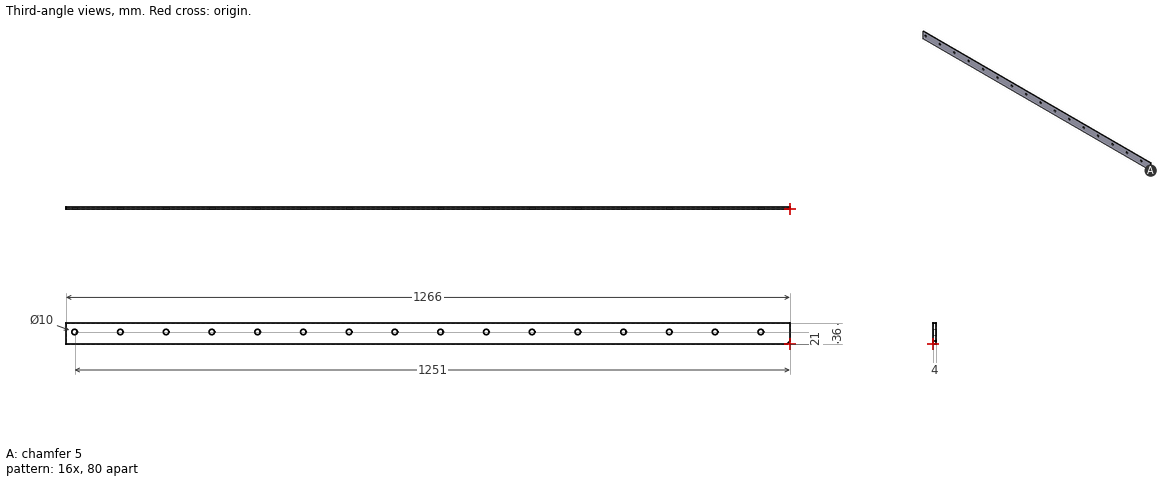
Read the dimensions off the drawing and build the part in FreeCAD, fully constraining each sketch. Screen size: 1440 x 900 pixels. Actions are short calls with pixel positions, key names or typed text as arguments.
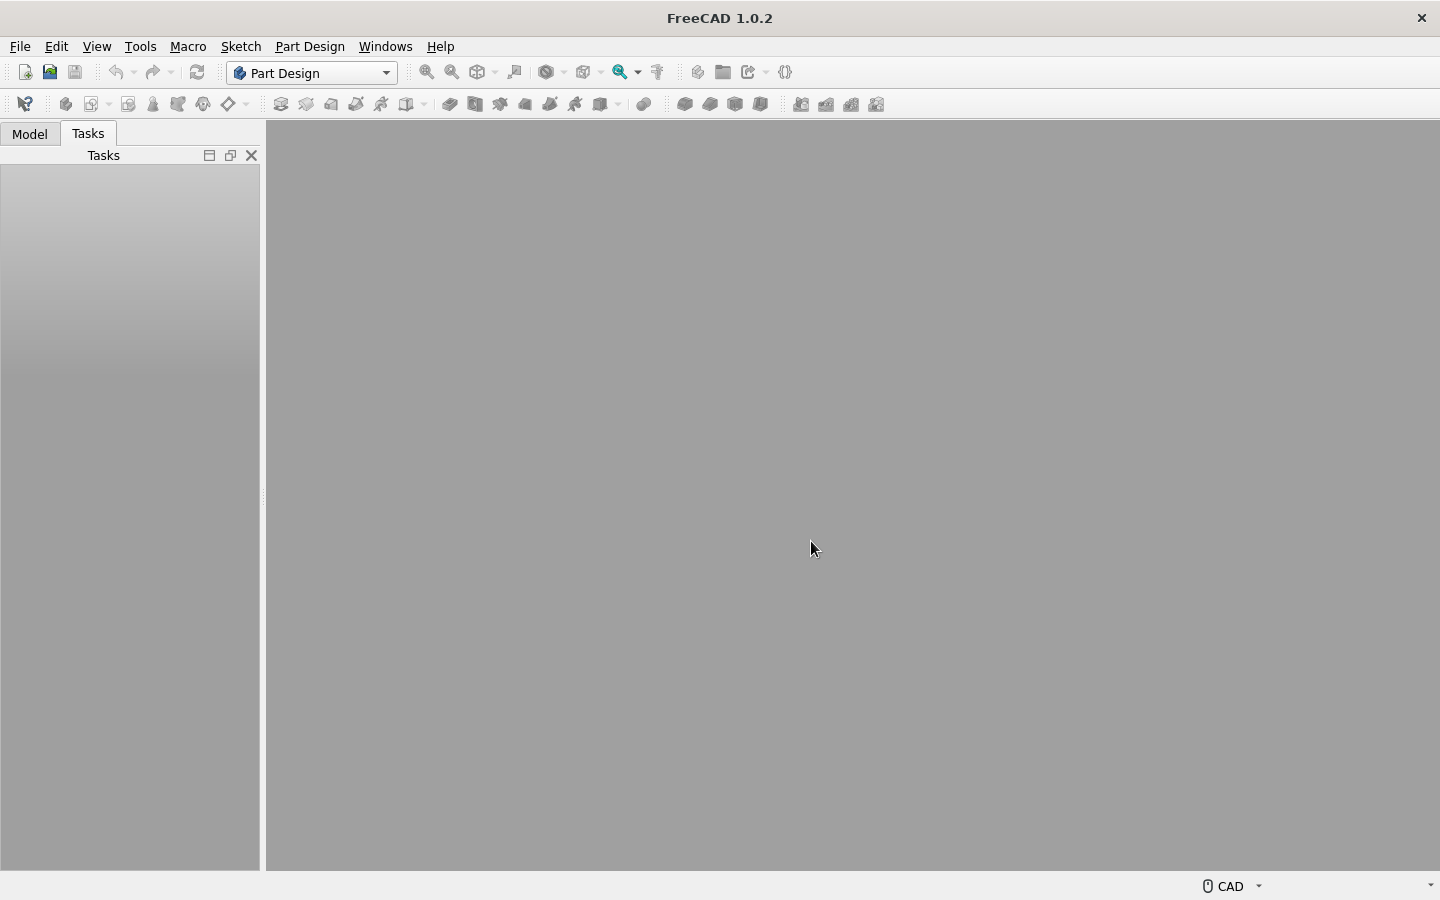
click(25, 72)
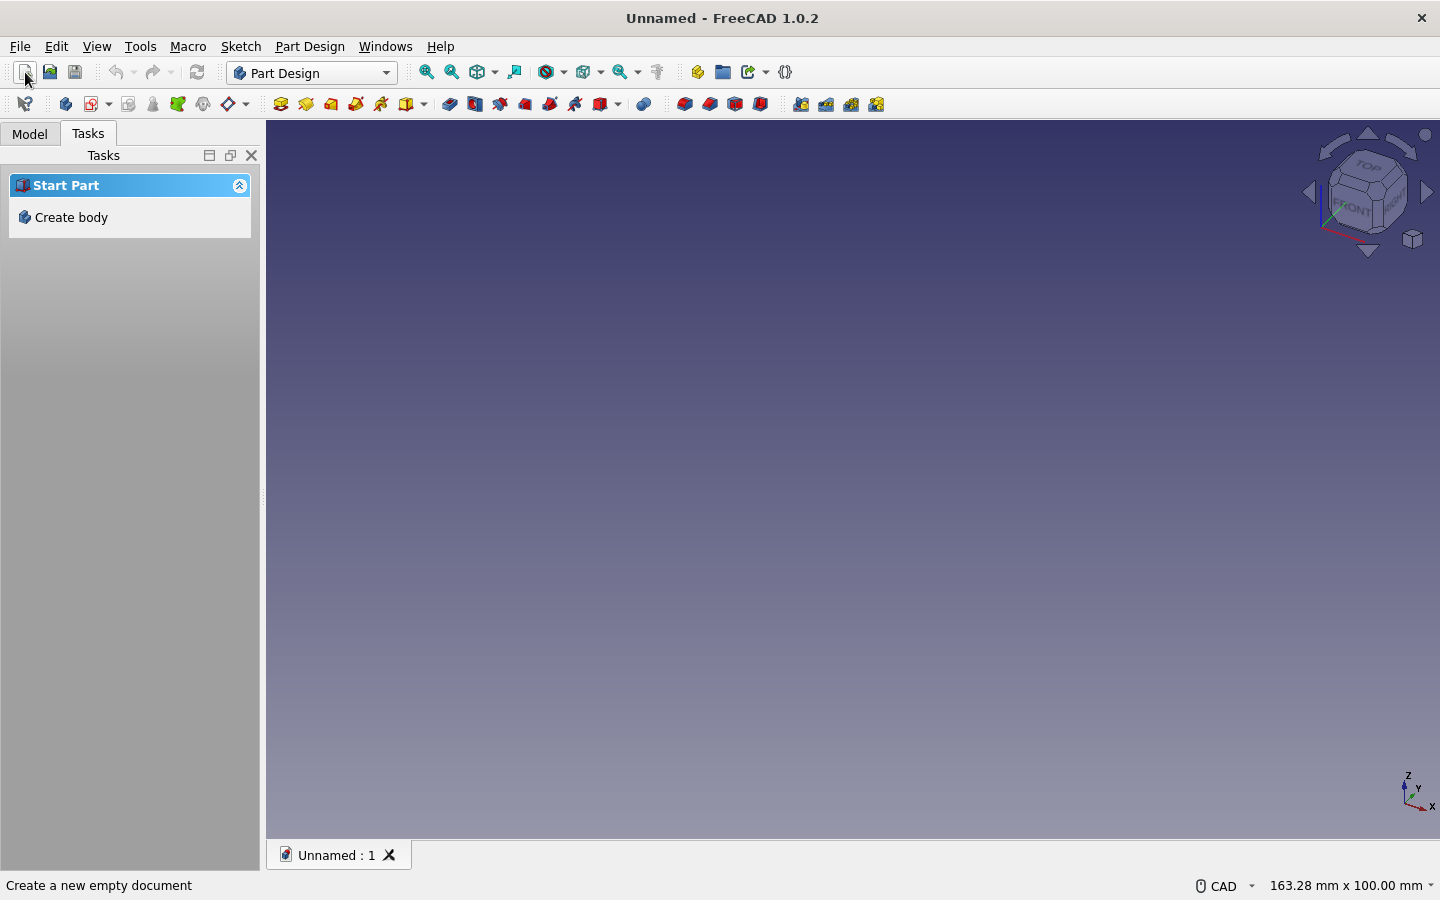
click(90, 104)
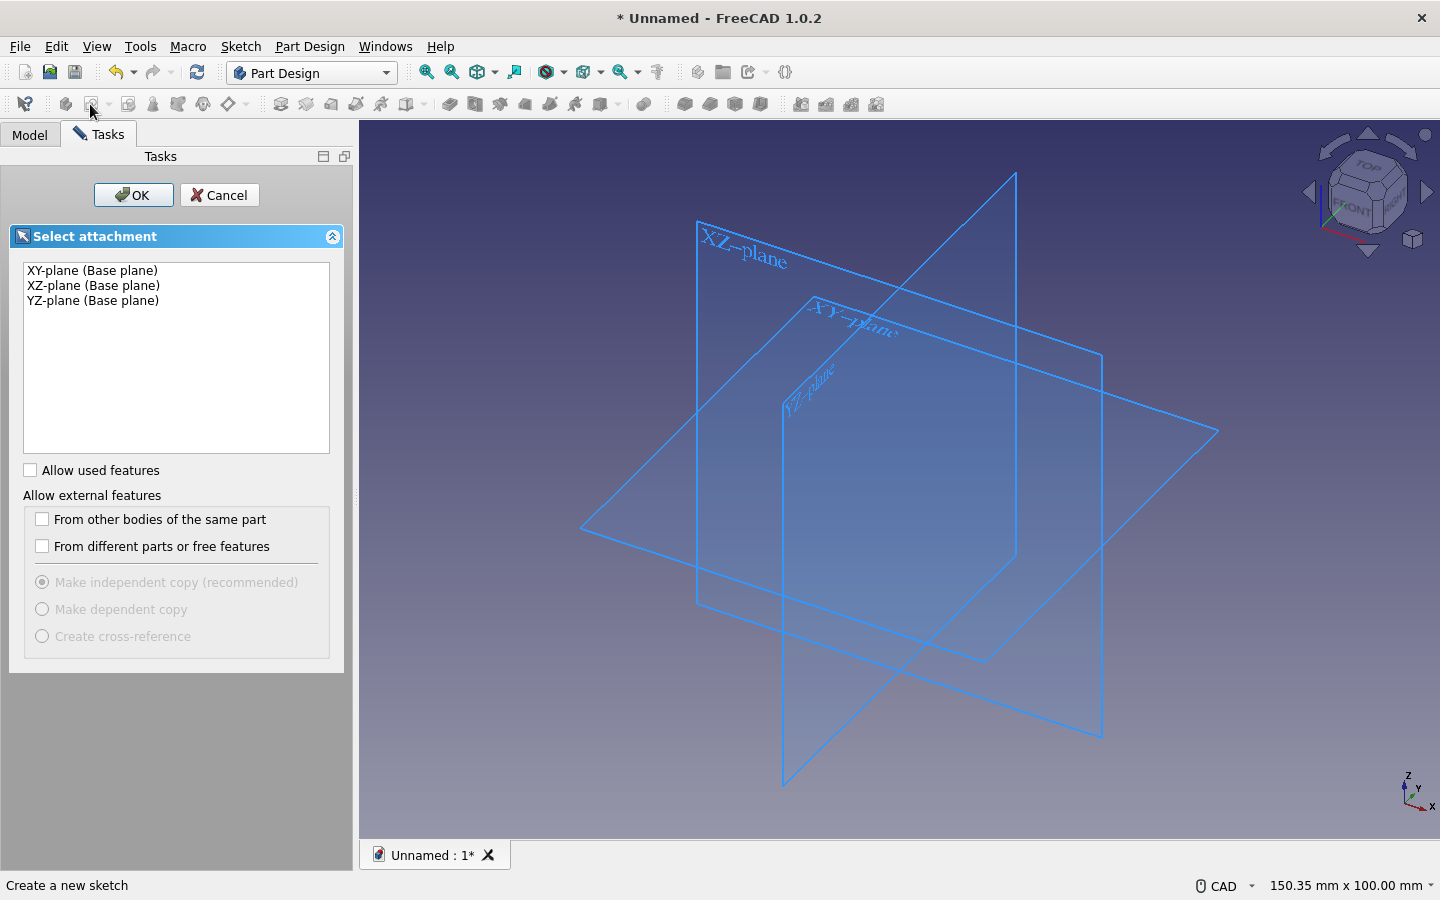
click(84, 286)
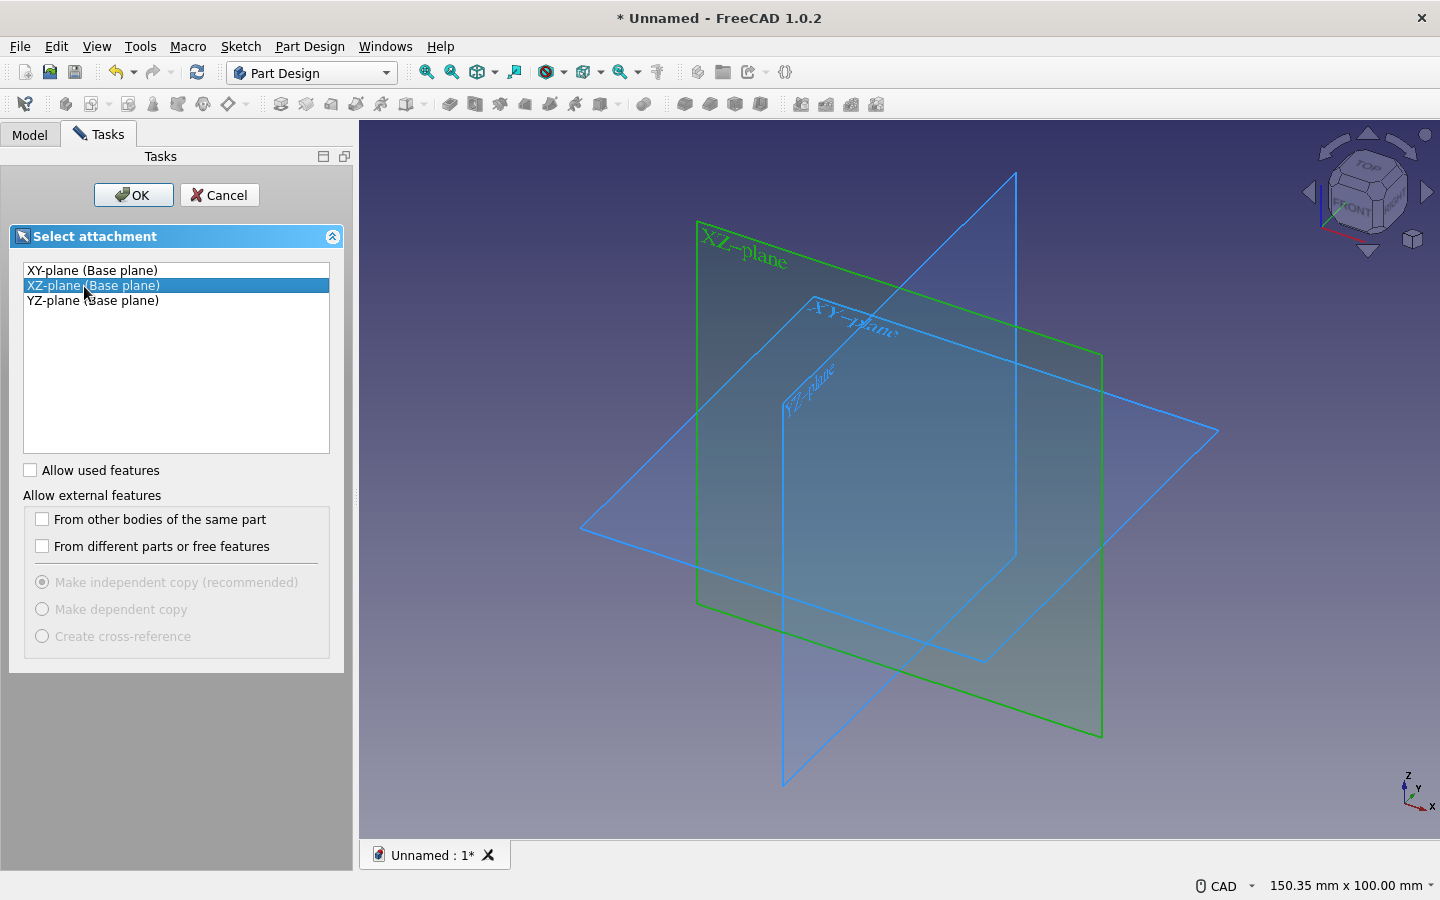
click(134, 195)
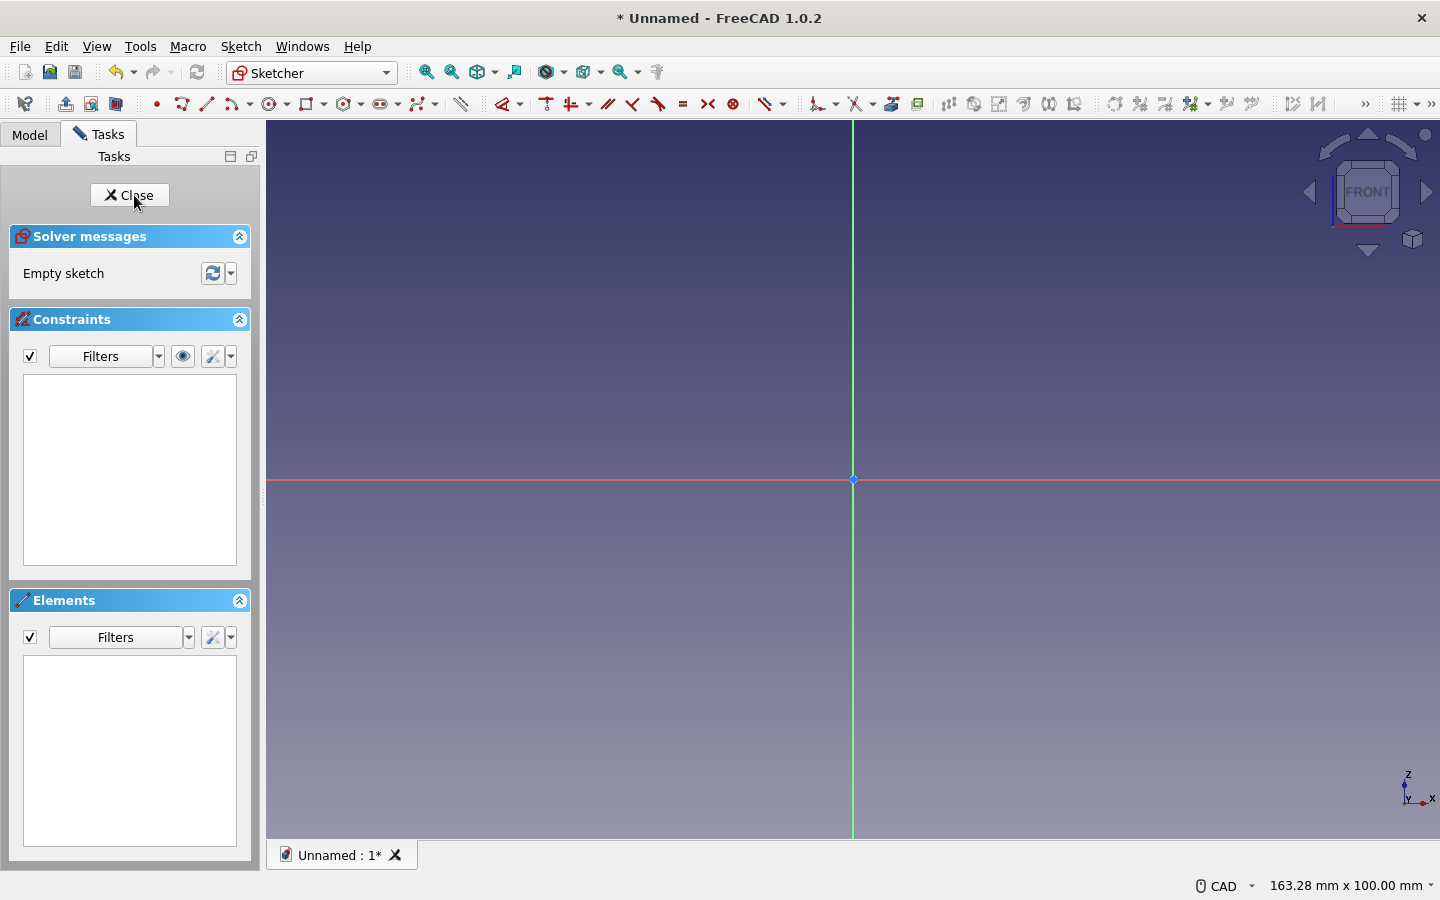
scroll(1144, 490, down, 13)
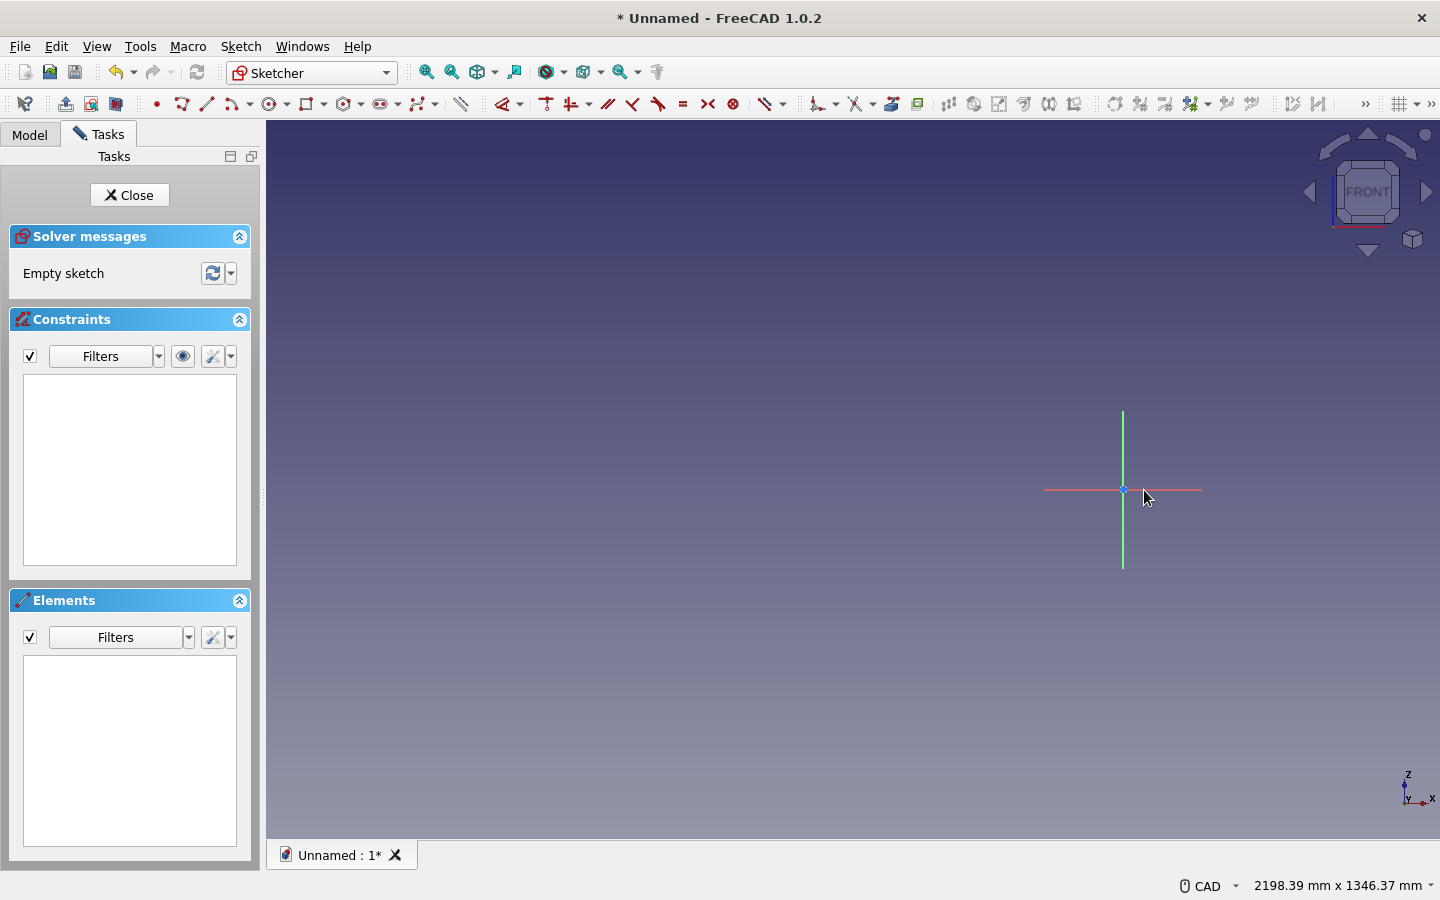
click(306, 104)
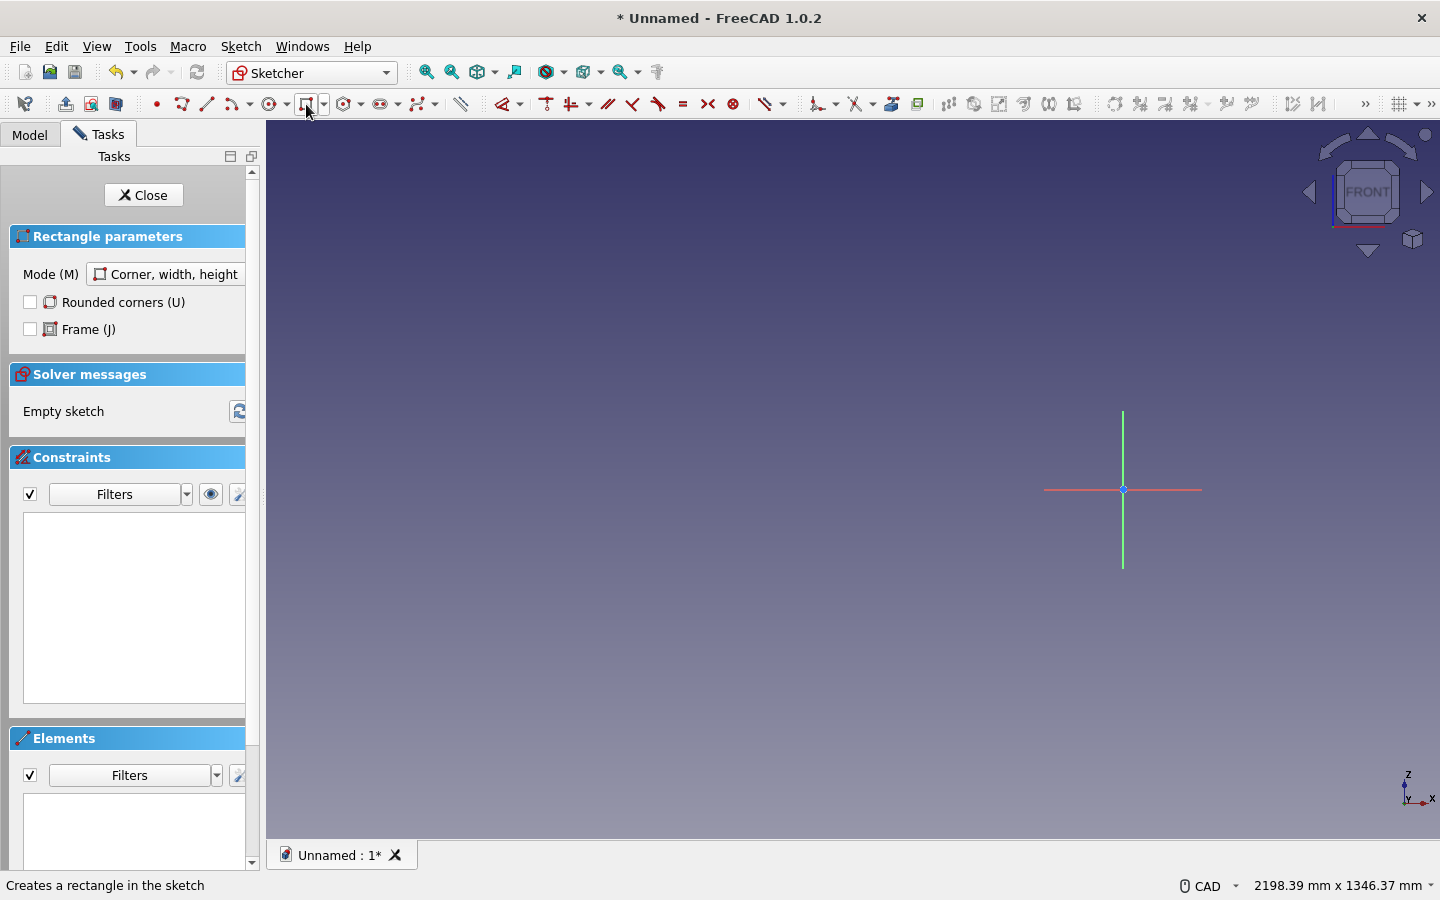
click(1123, 490)
click(447, 470)
key(Escape)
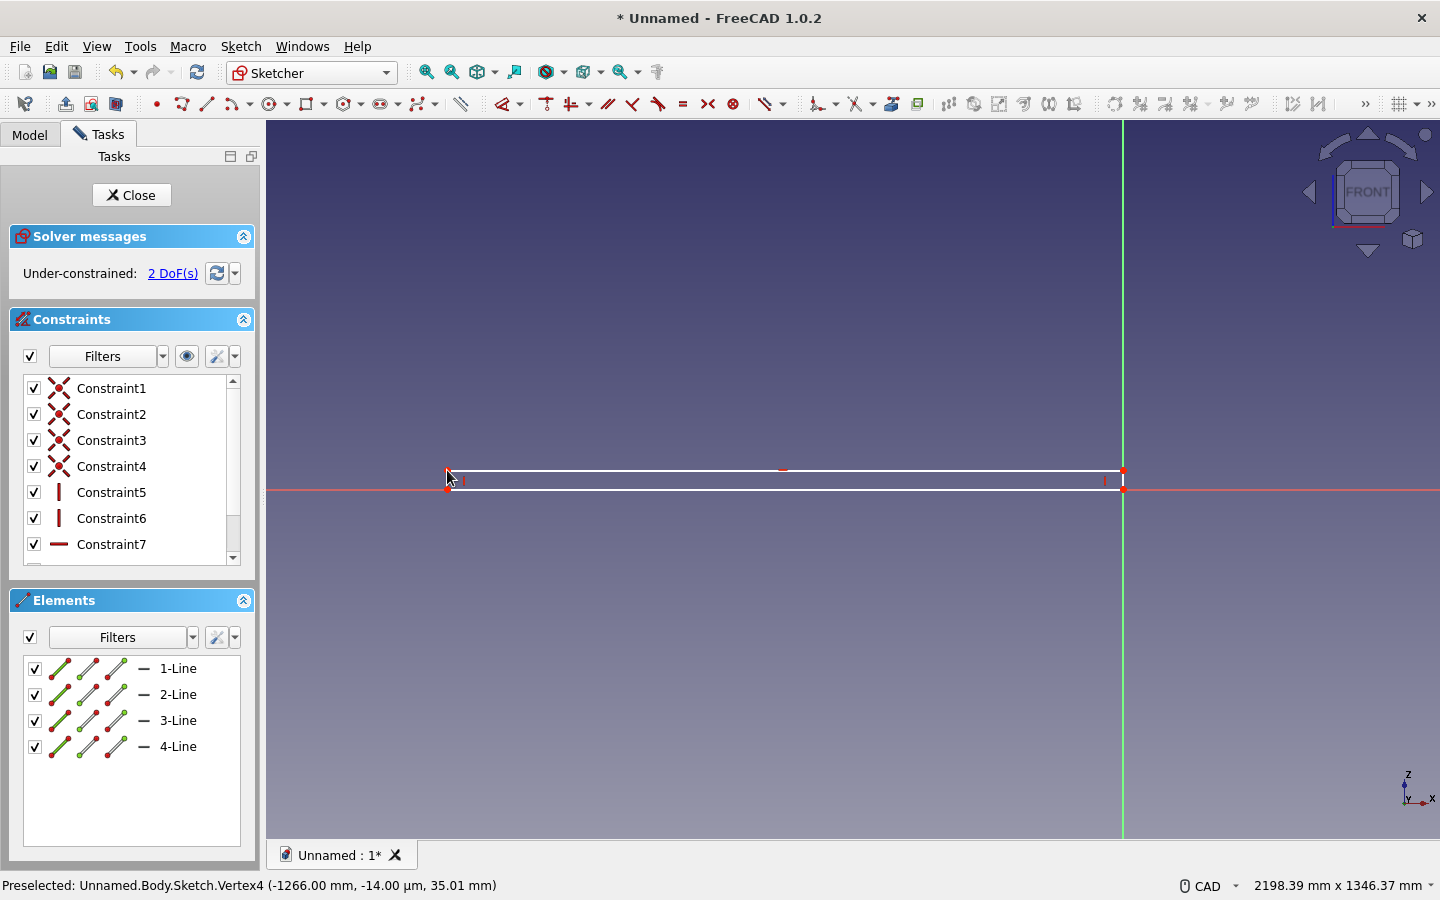
scroll(1123, 480, up, 4)